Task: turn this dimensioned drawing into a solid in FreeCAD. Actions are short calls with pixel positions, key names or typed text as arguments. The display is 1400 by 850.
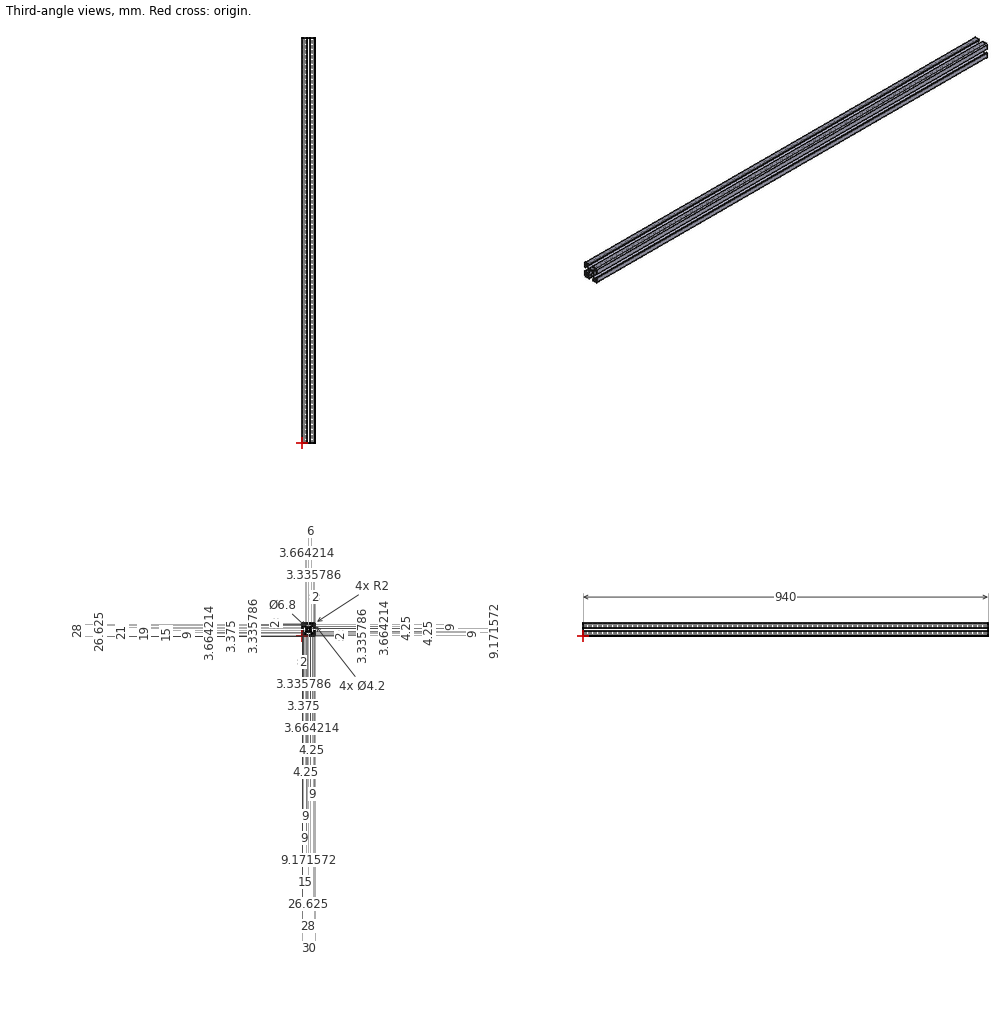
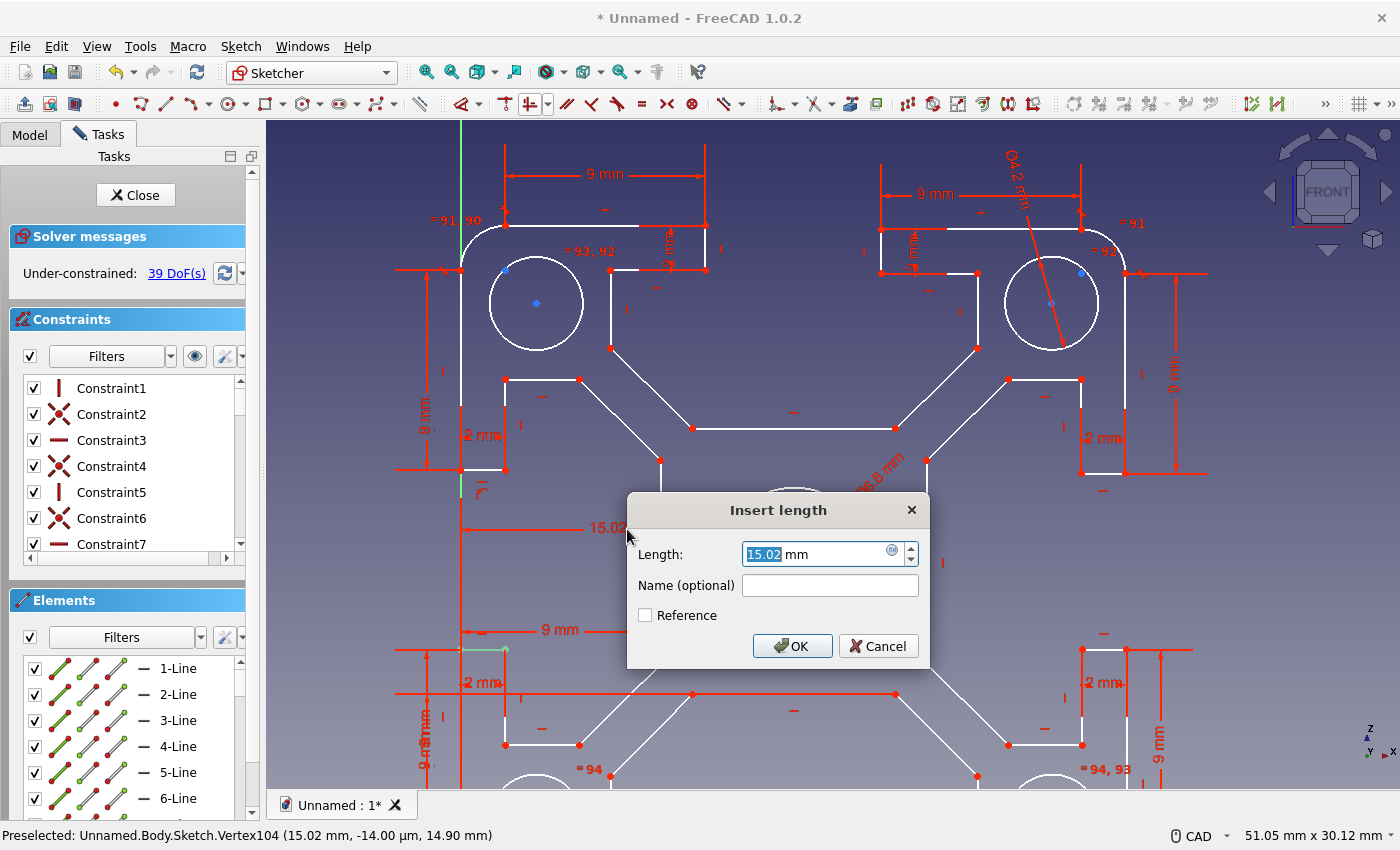
text(15)
key(Return)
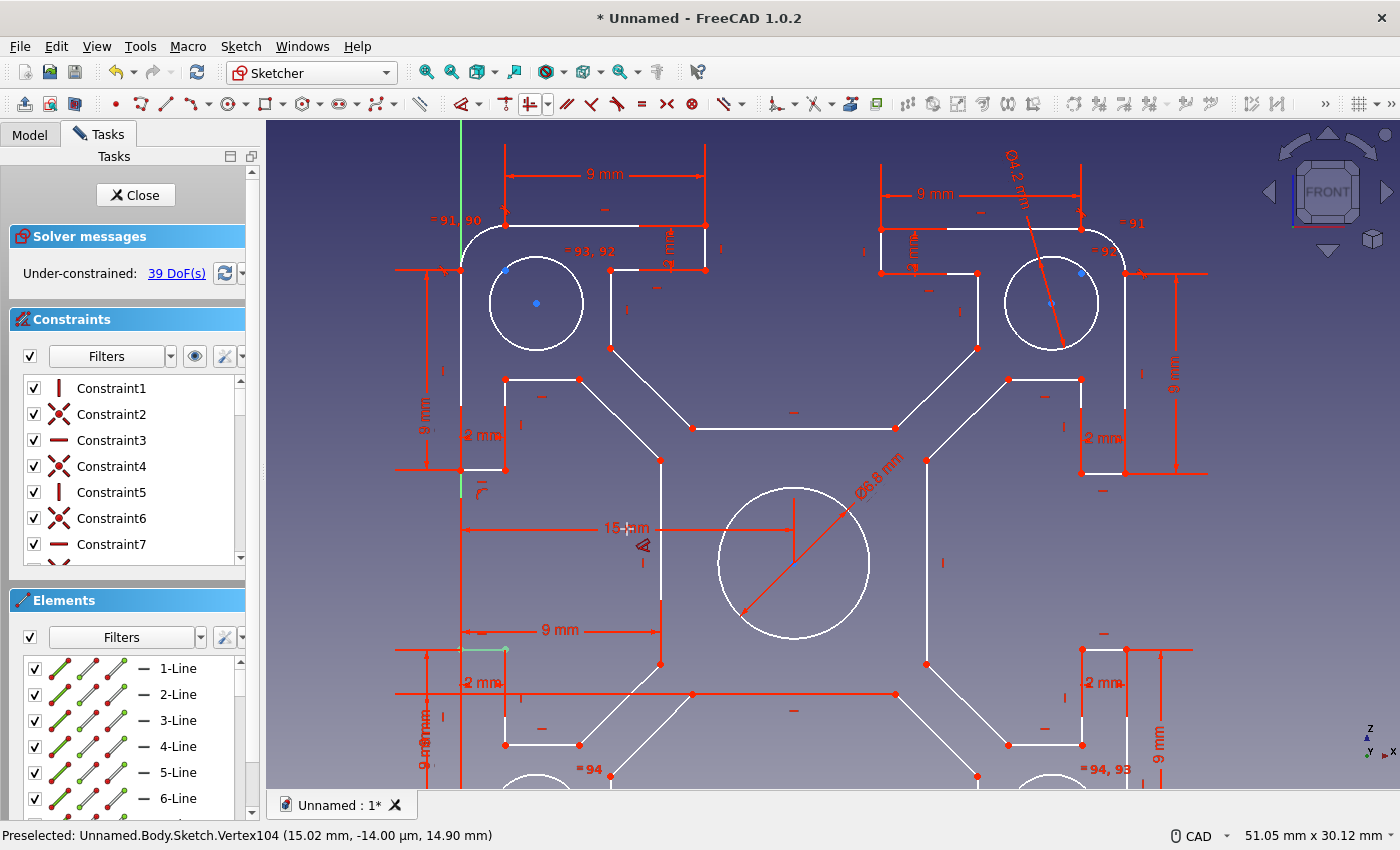
click(794, 563)
click(427, 662)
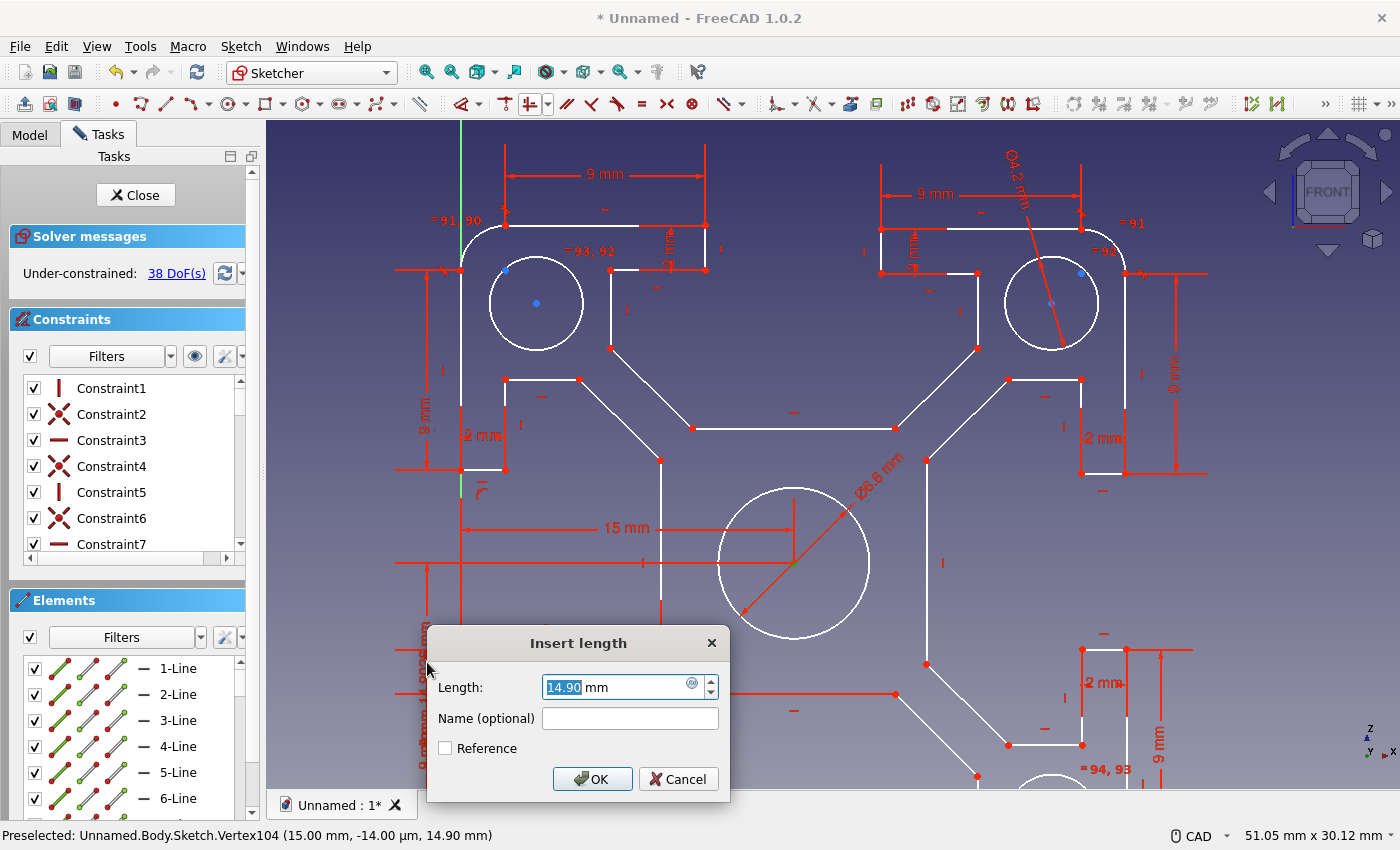
text(15)
key(Return)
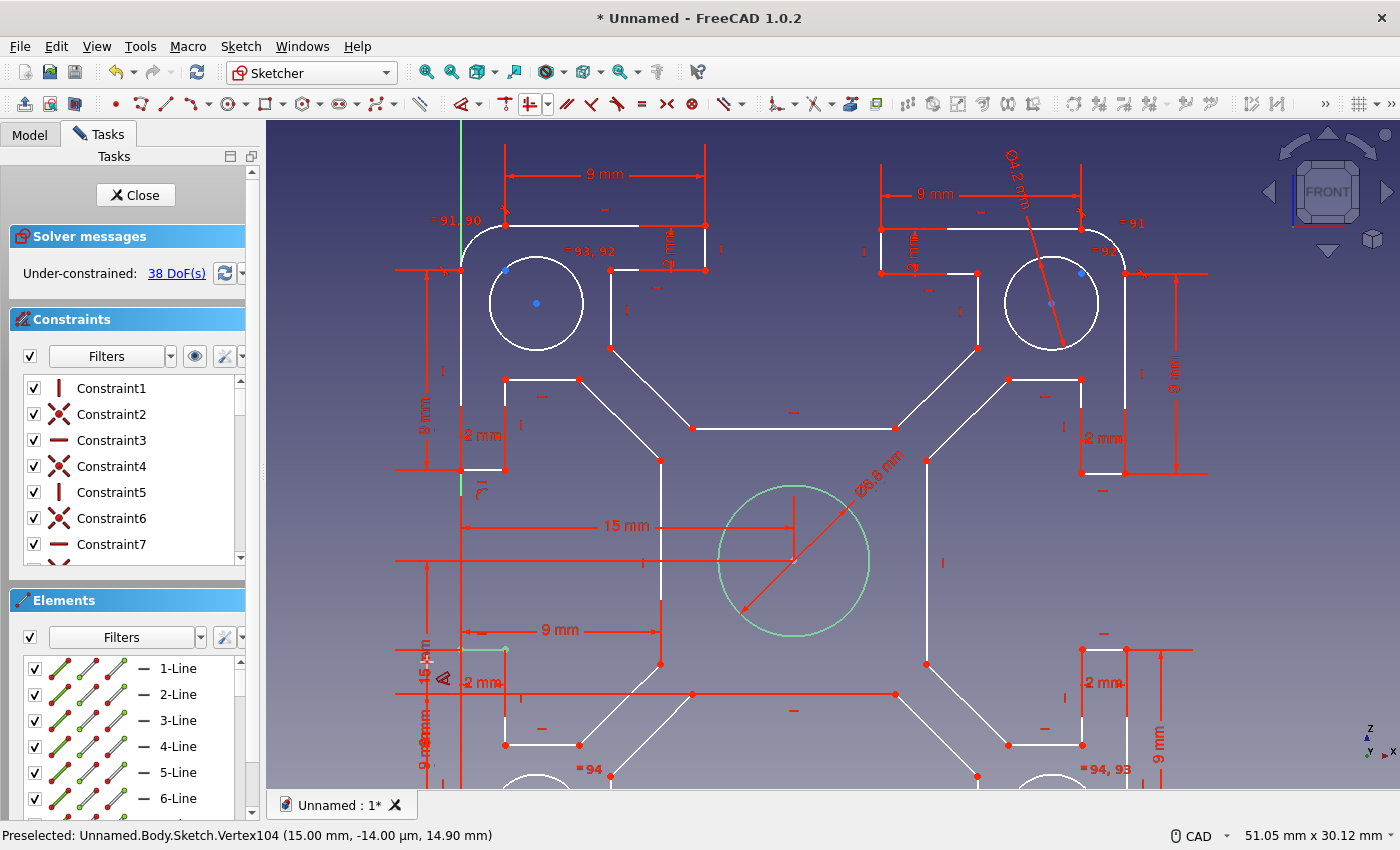
click(927, 460)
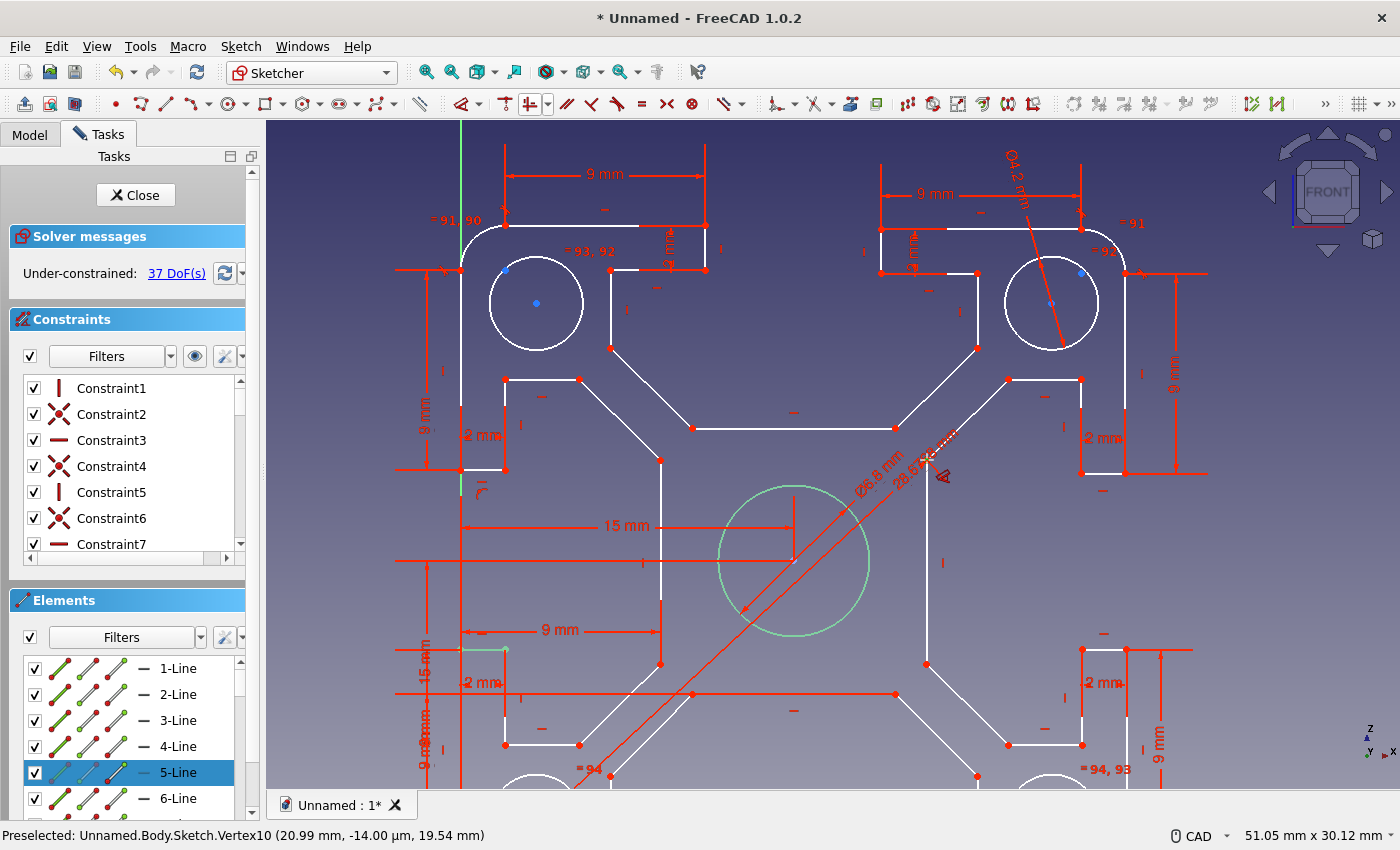
click(794, 561)
click(830, 595)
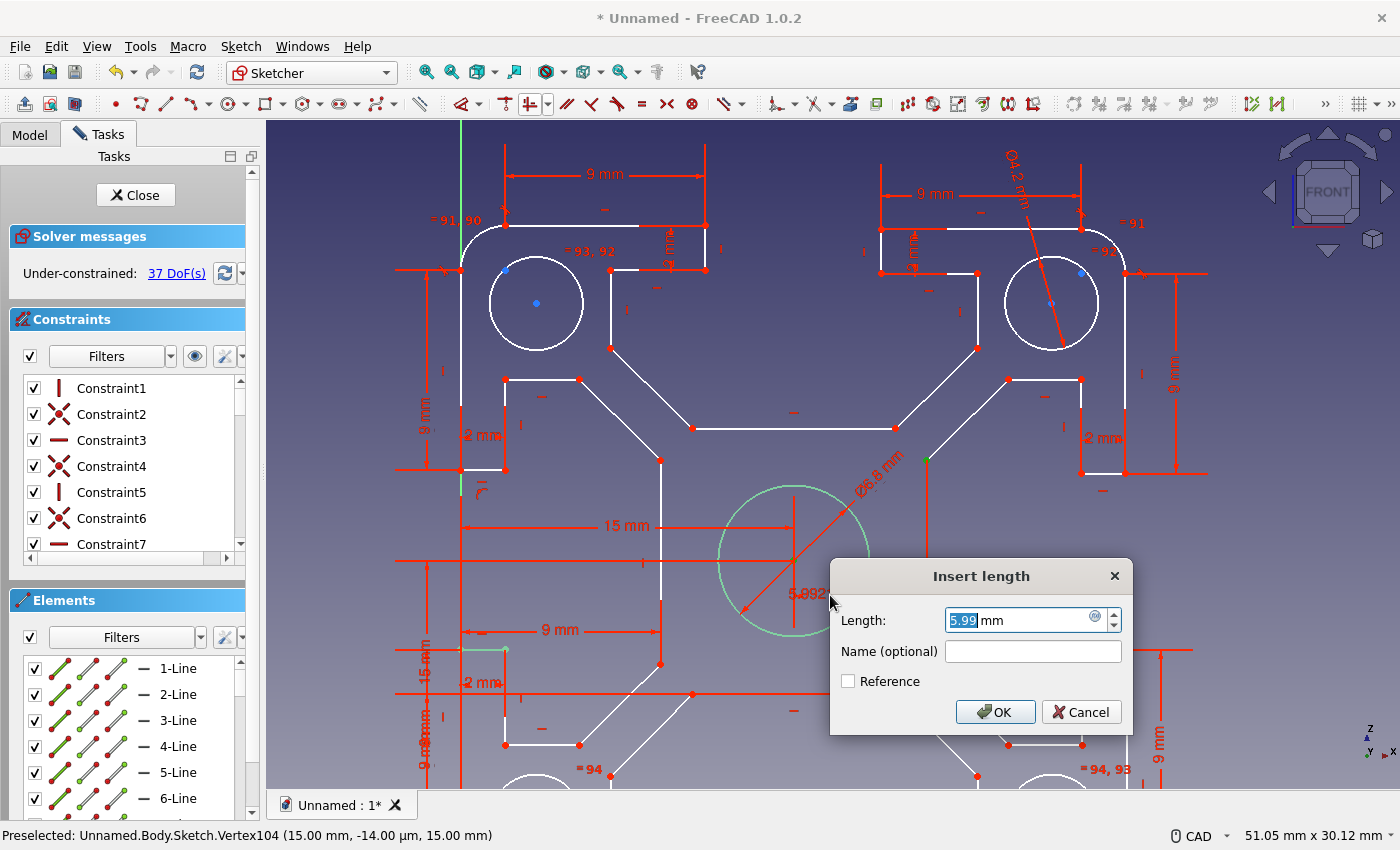
text(6)
key(Return)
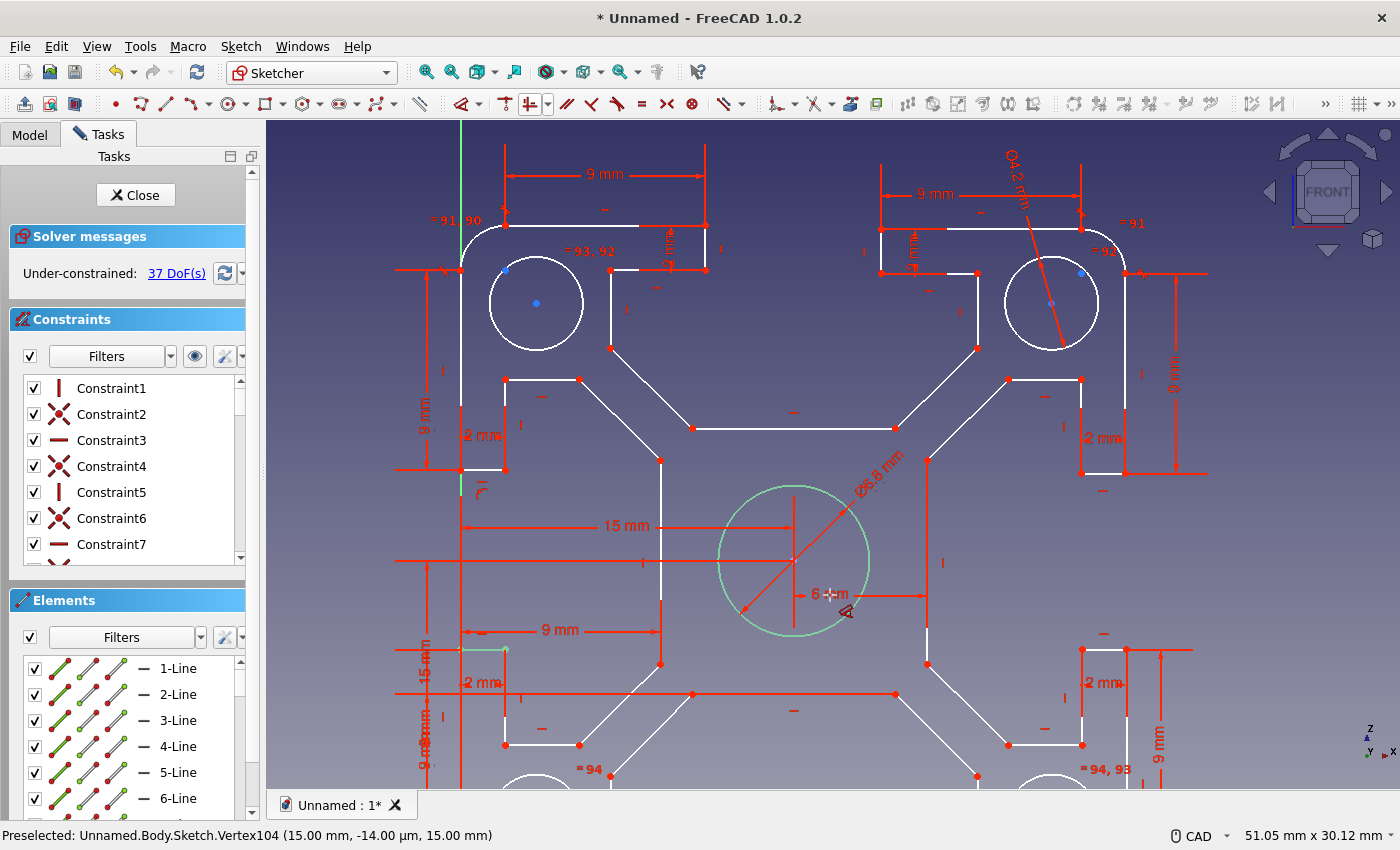
click(1125, 274)
click(793, 240)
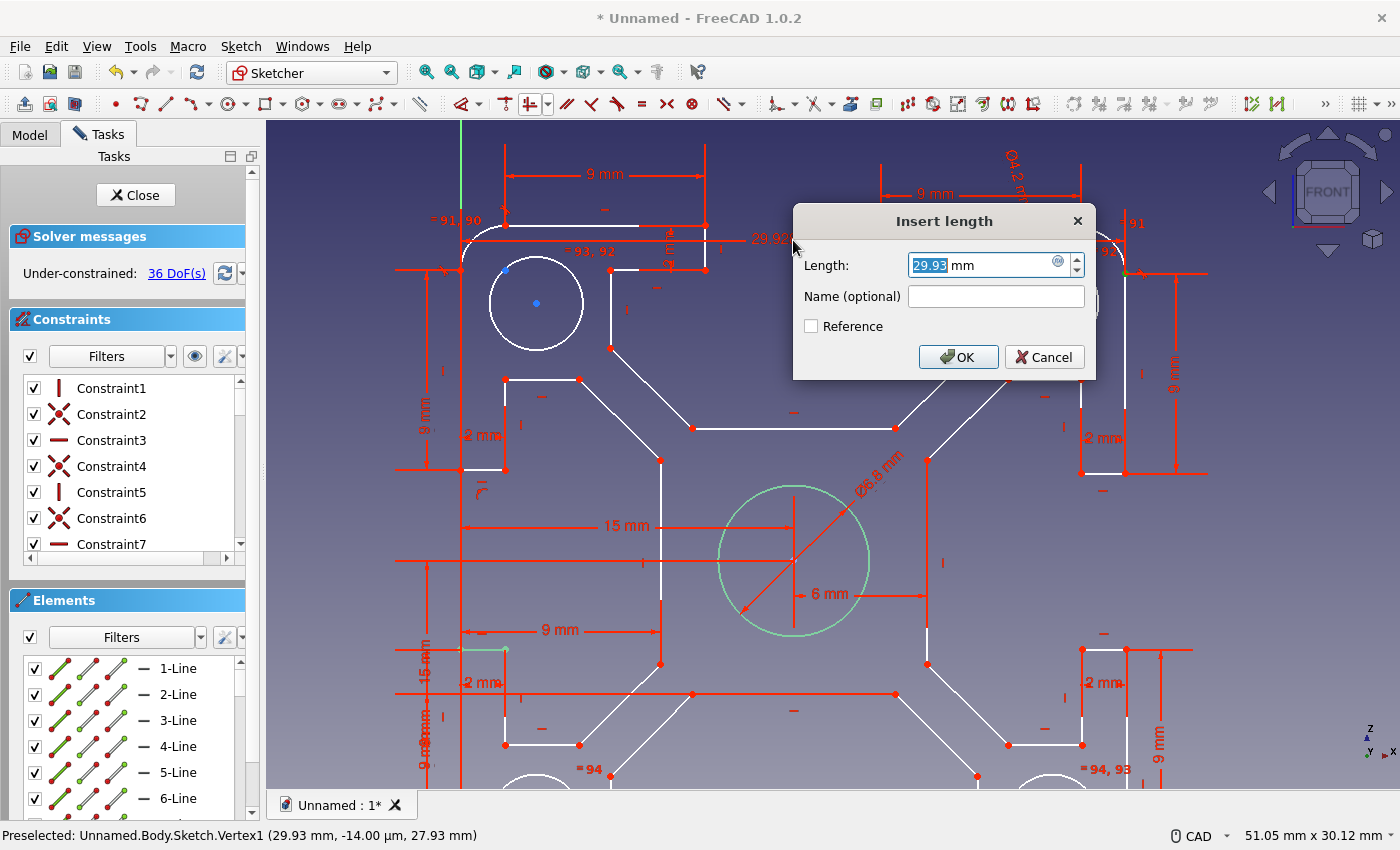
text(30)
key(Return)